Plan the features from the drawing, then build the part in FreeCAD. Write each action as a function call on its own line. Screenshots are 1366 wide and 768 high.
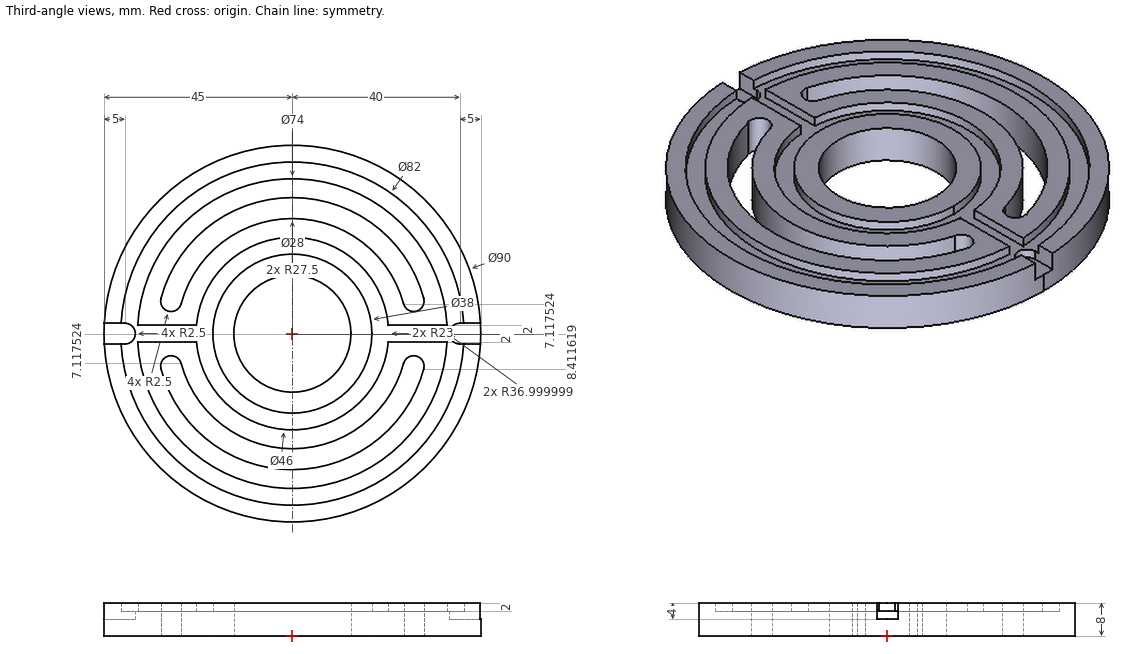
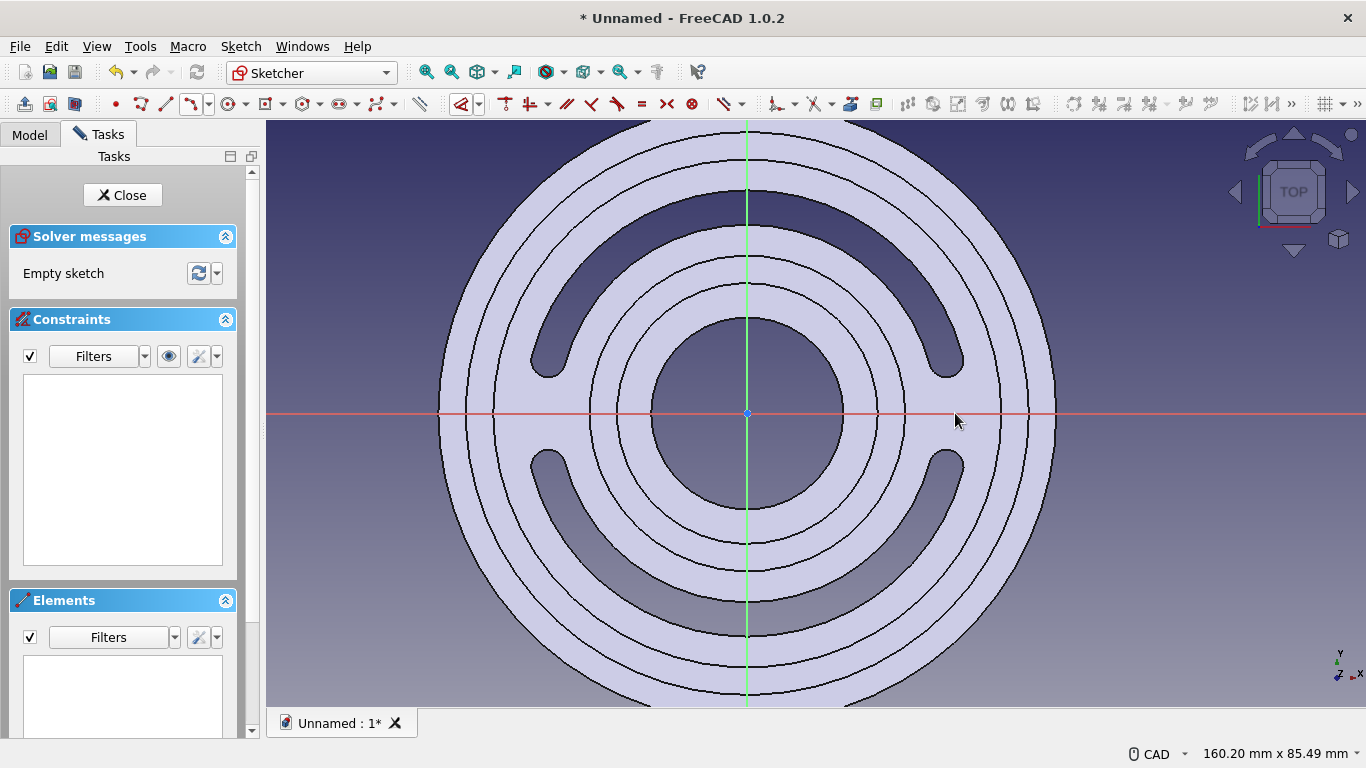
scroll(438, 414, up, 2)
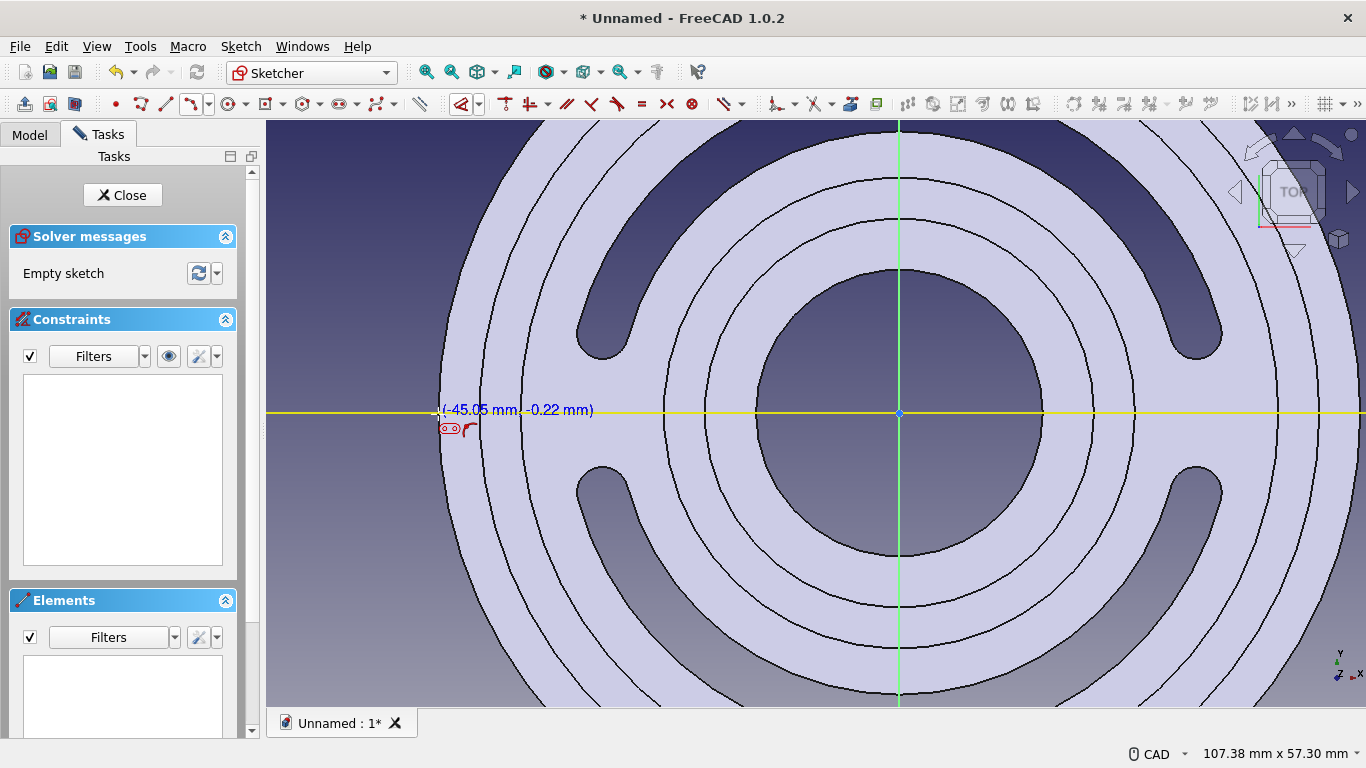
click(438, 413)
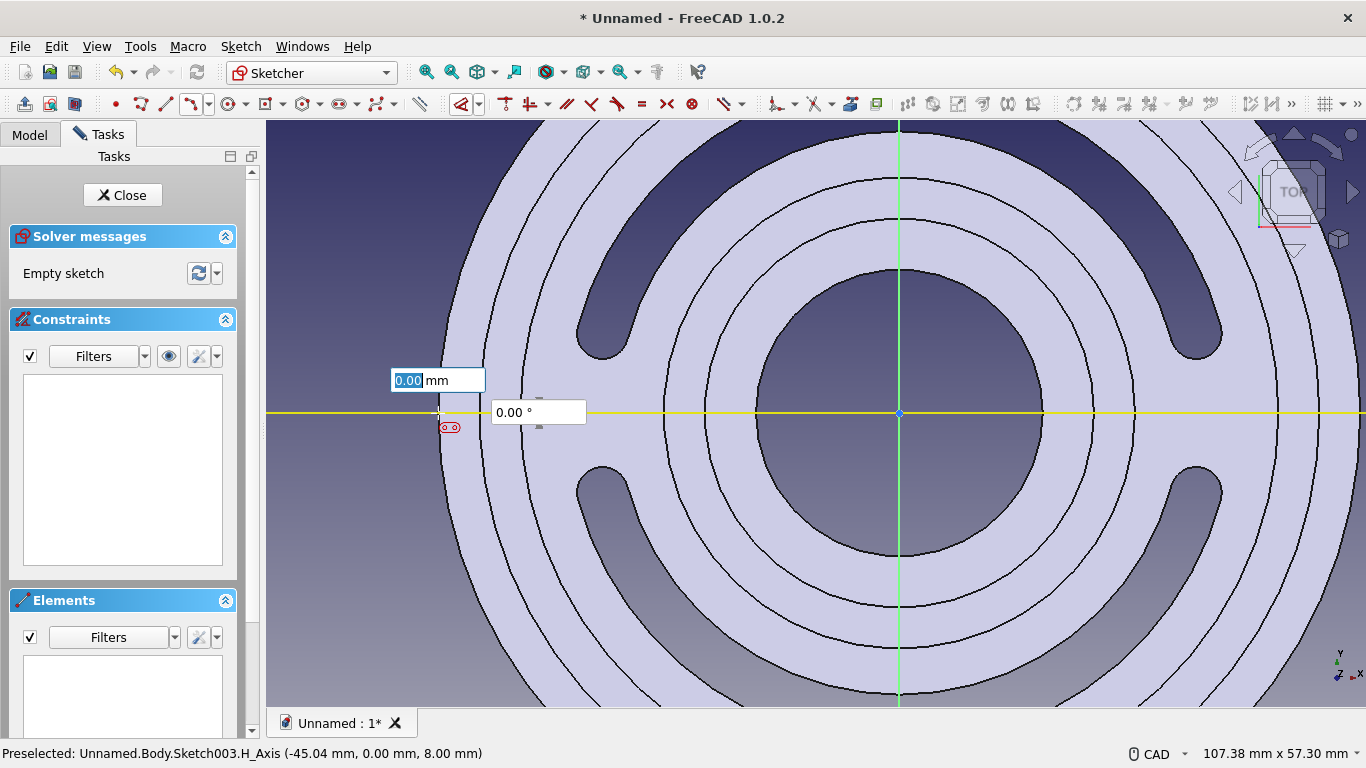
click(490, 404)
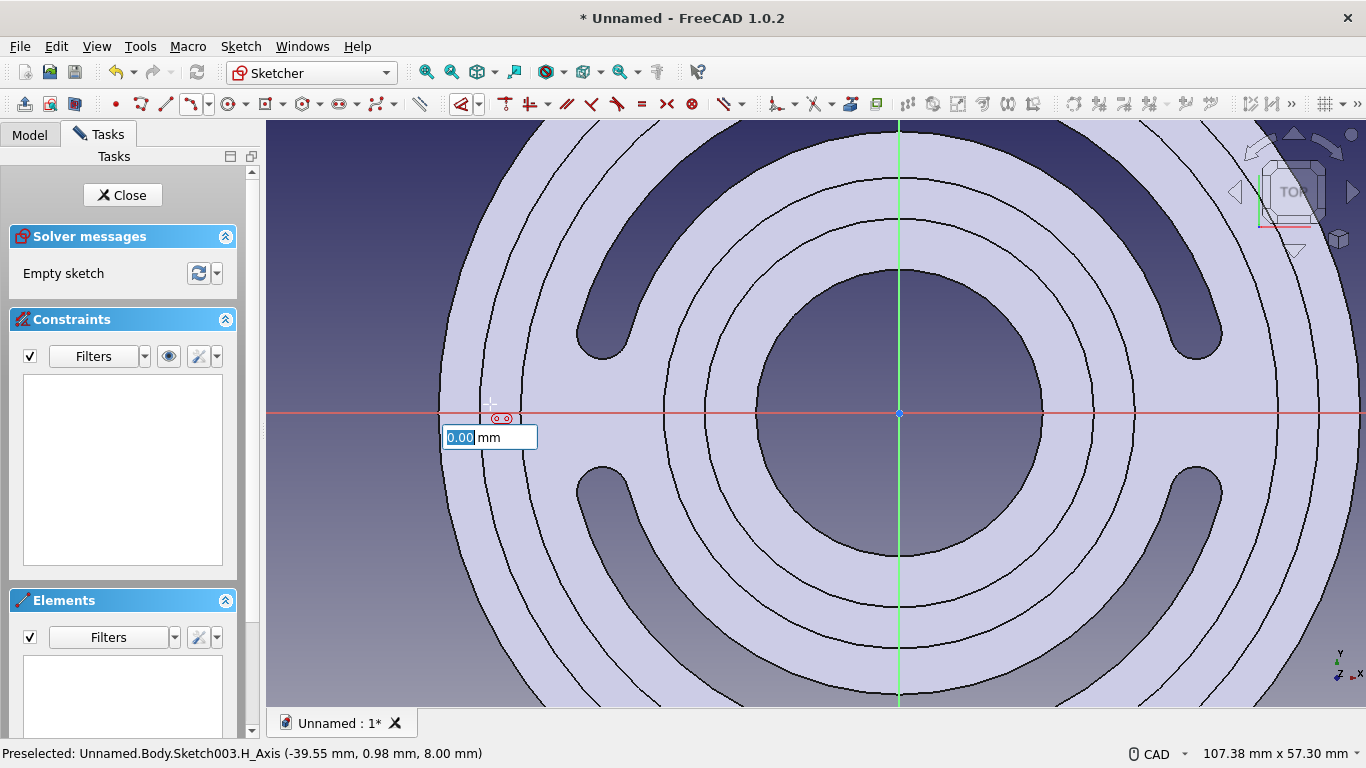
click(464, 439)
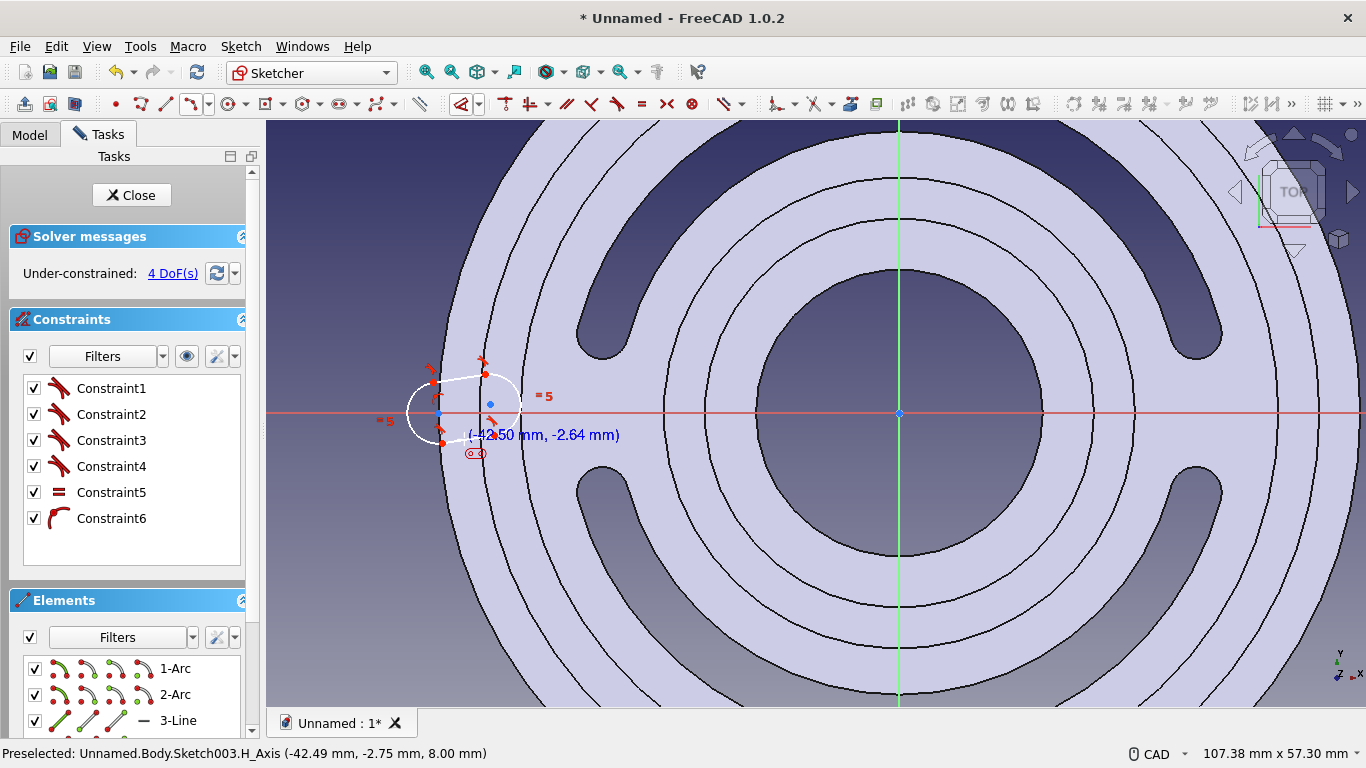
scroll(439, 415, down, 2)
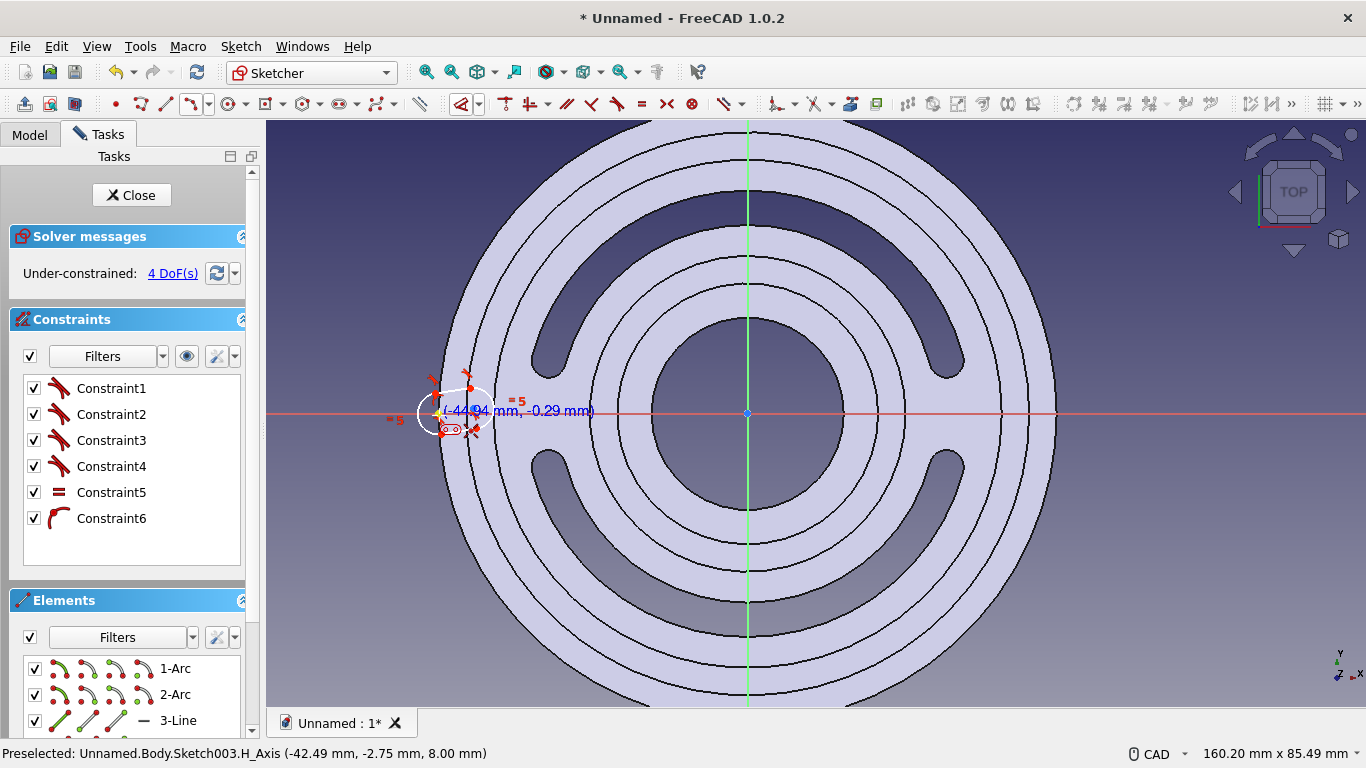
scroll(1022, 414, up, 2)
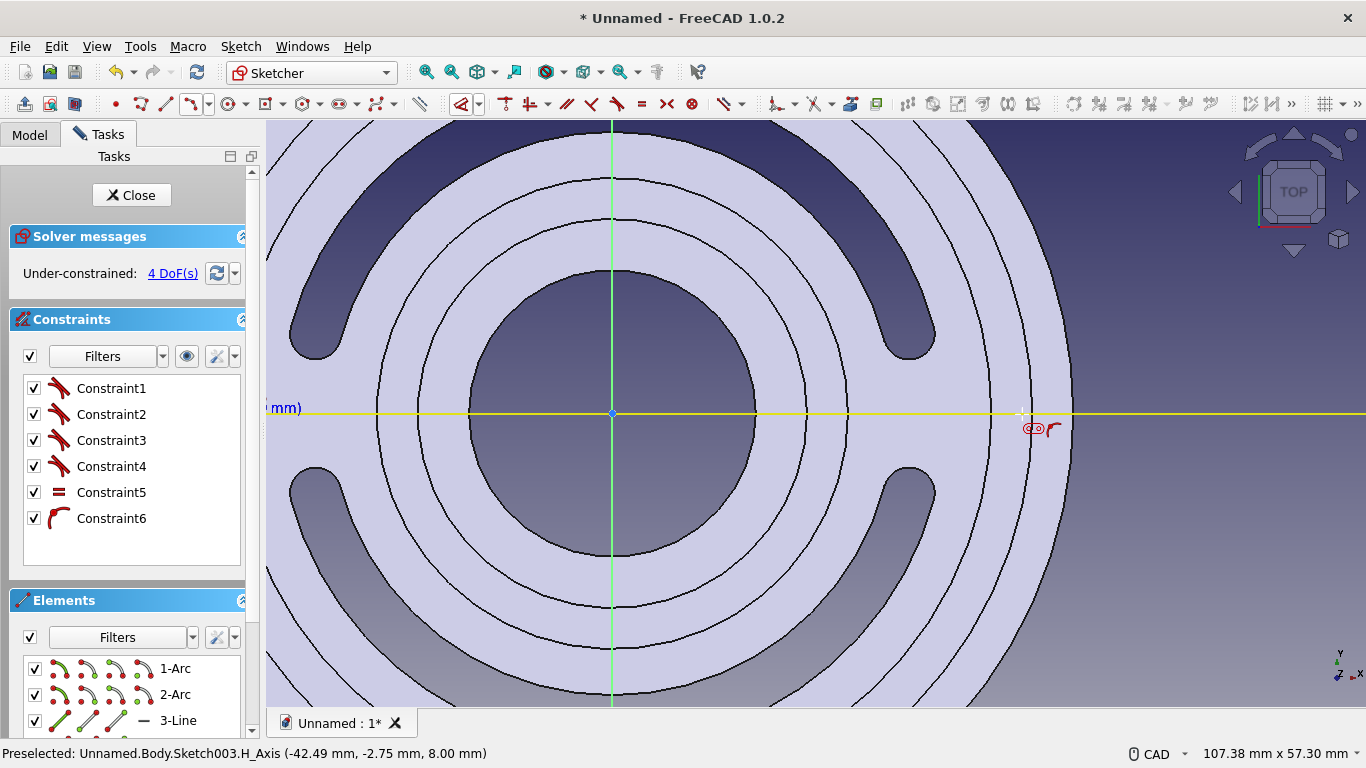
click(1022, 413)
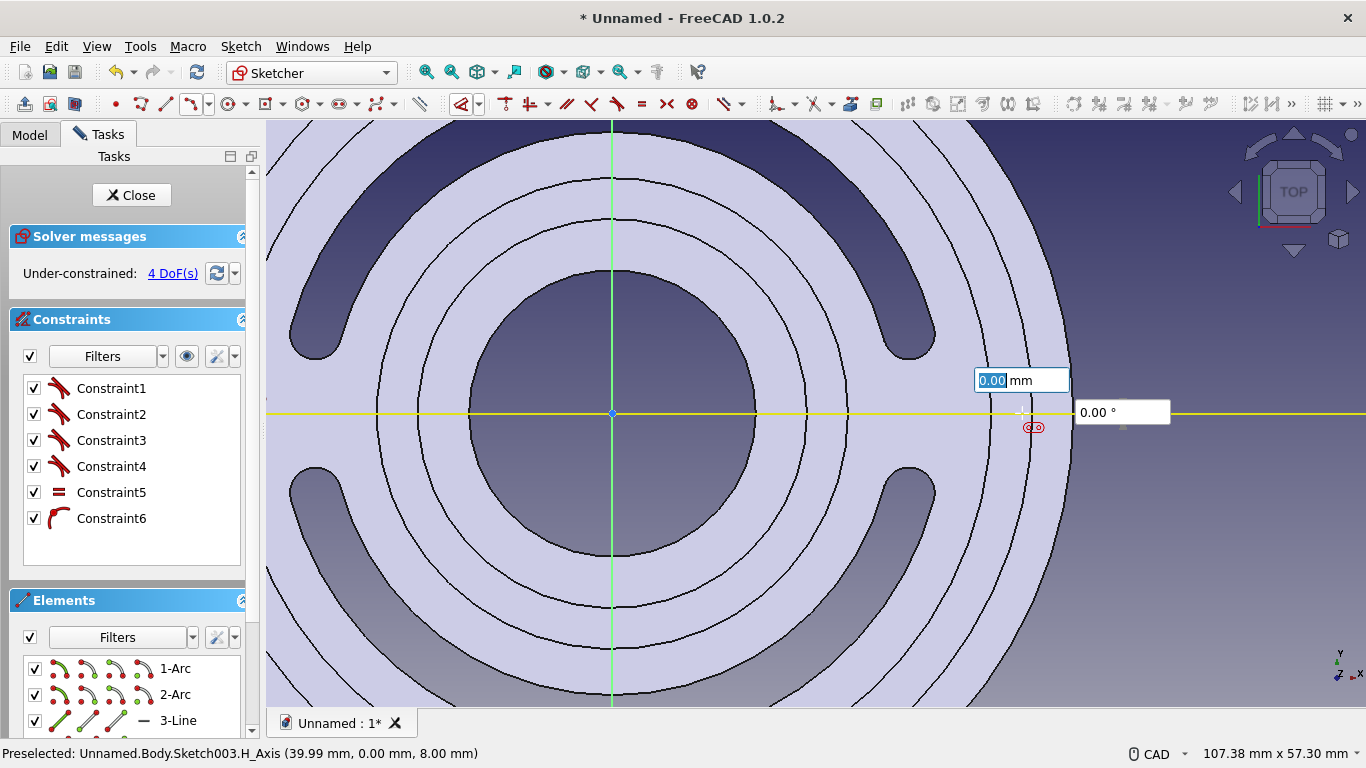
click(1073, 404)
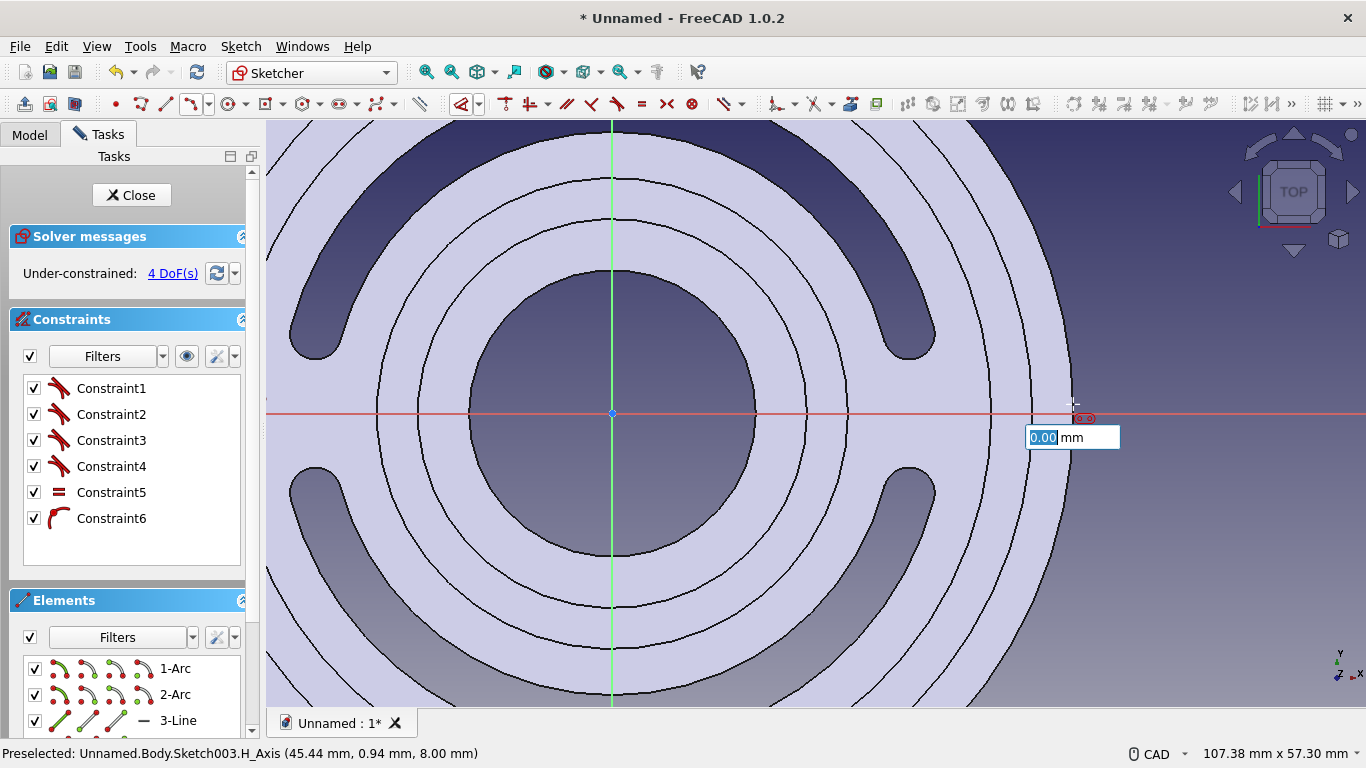
click(1048, 439)
key(Escape)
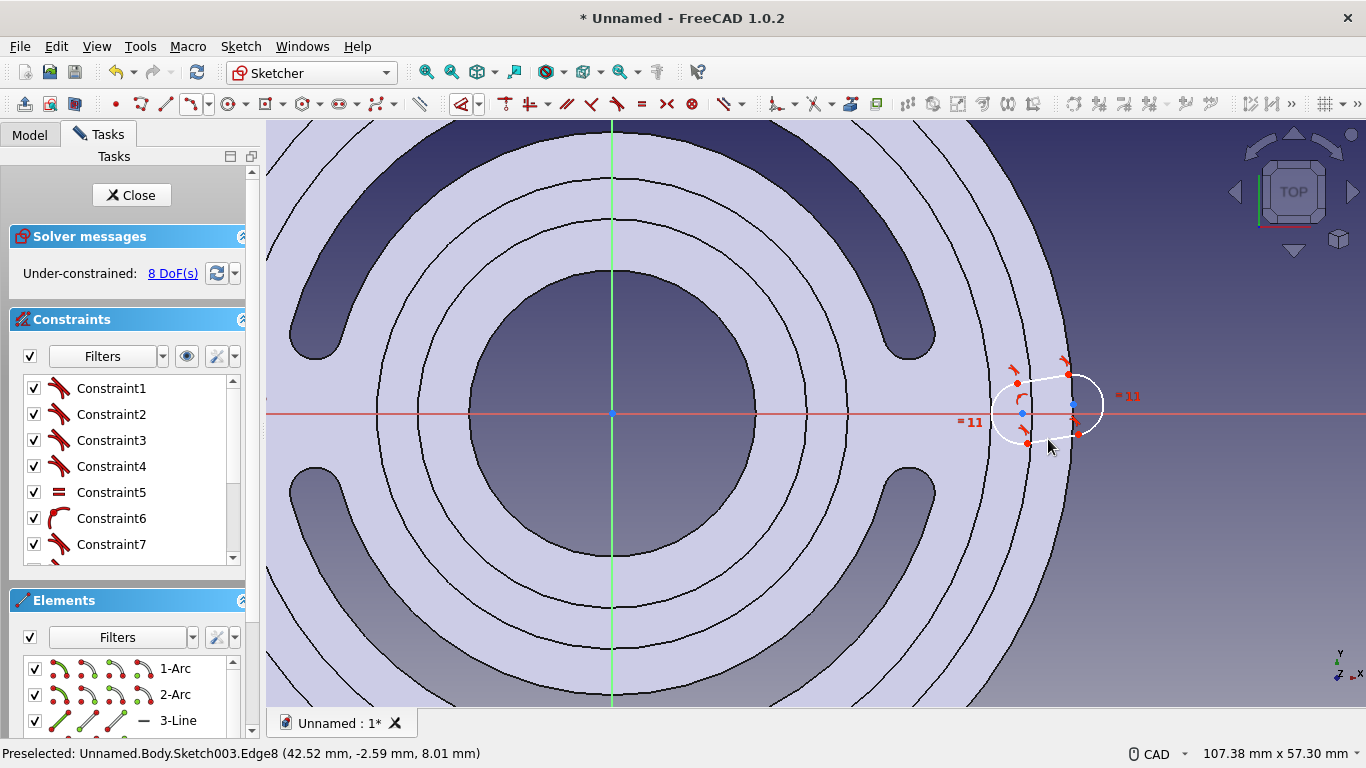
scroll(1022, 414, down, 2)